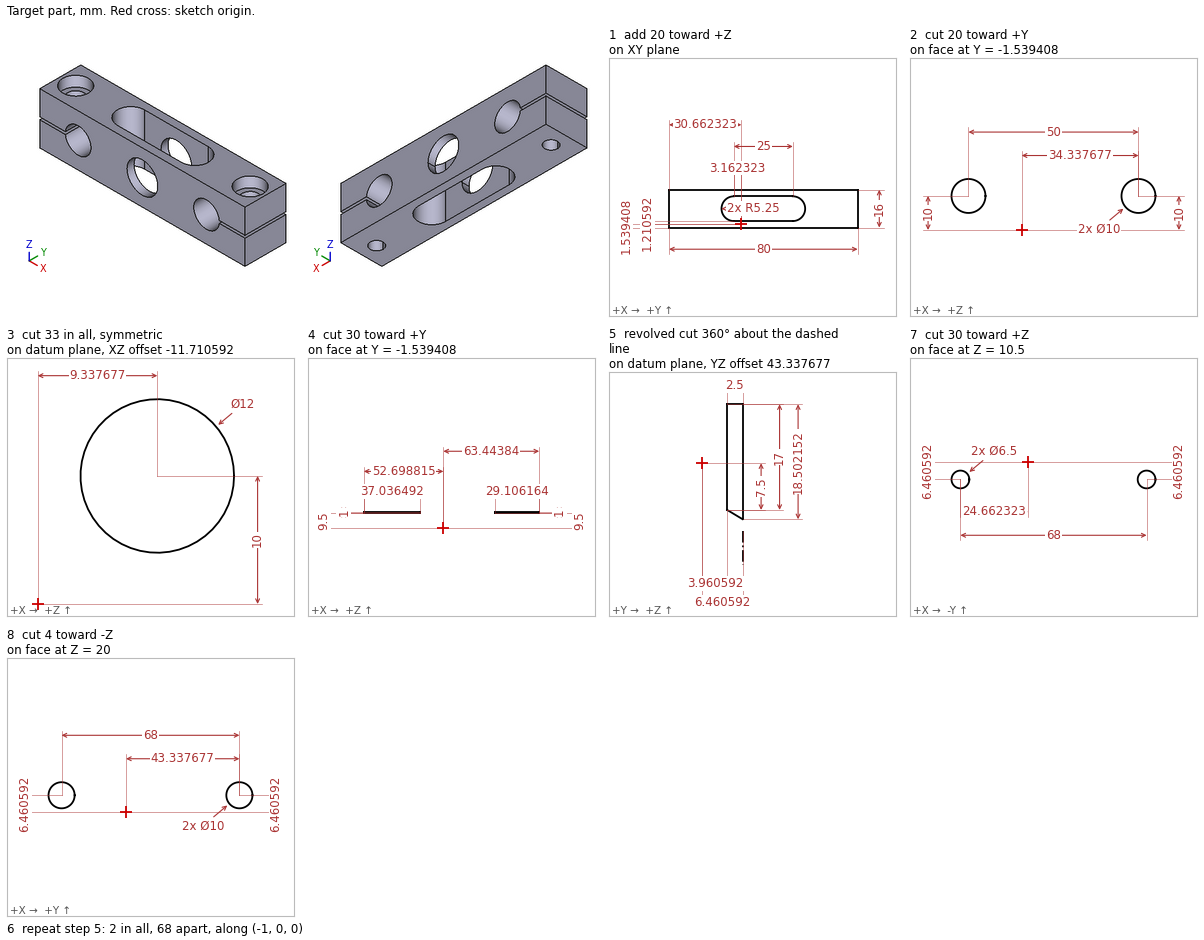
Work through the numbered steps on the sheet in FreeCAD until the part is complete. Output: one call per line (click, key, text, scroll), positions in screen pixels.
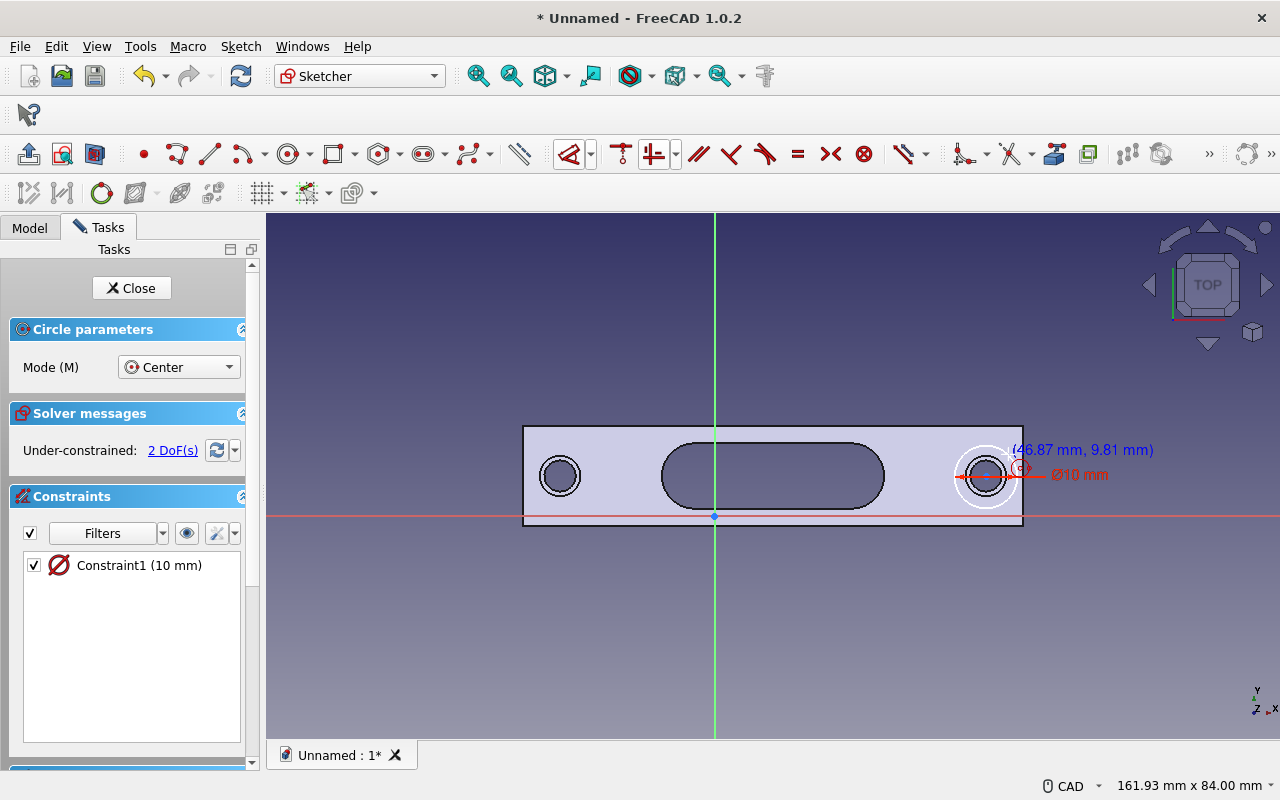
click(560, 476)
move(582, 454)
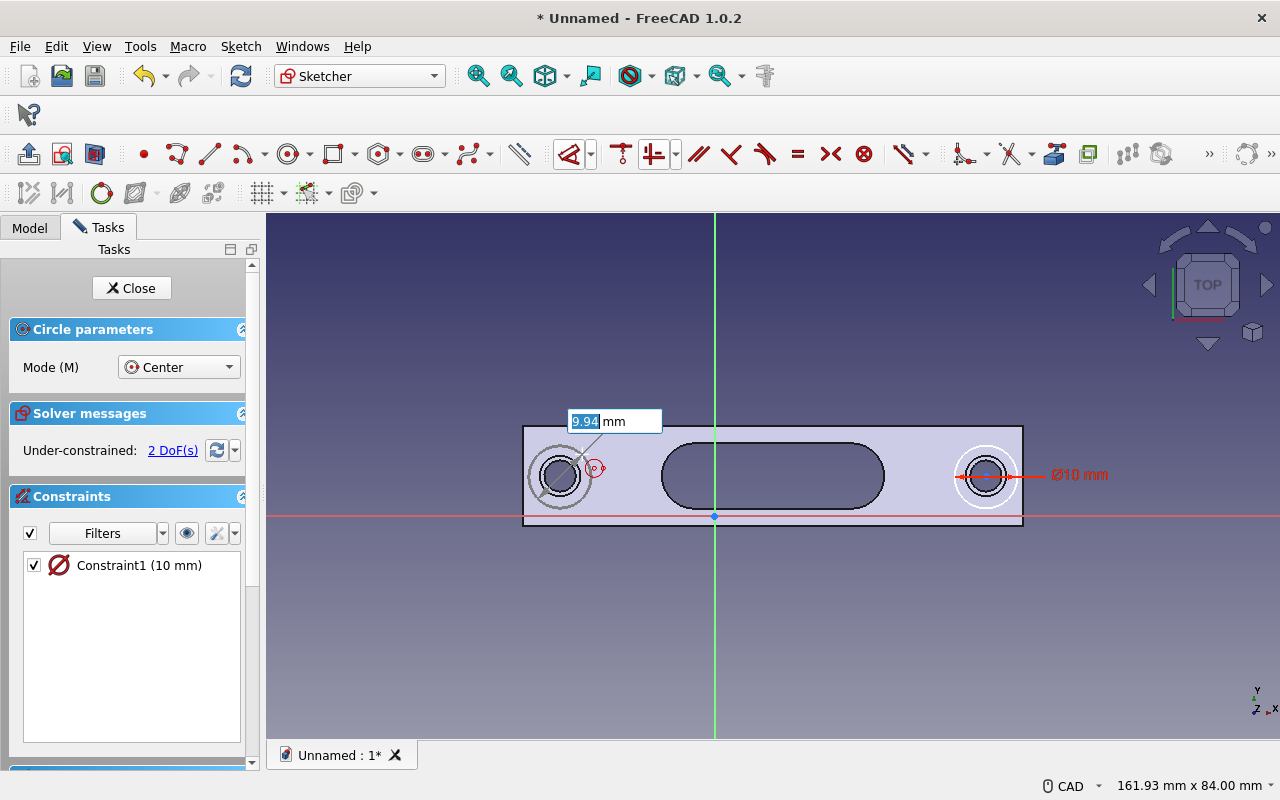
text(10)
key(Return)
key(Escape)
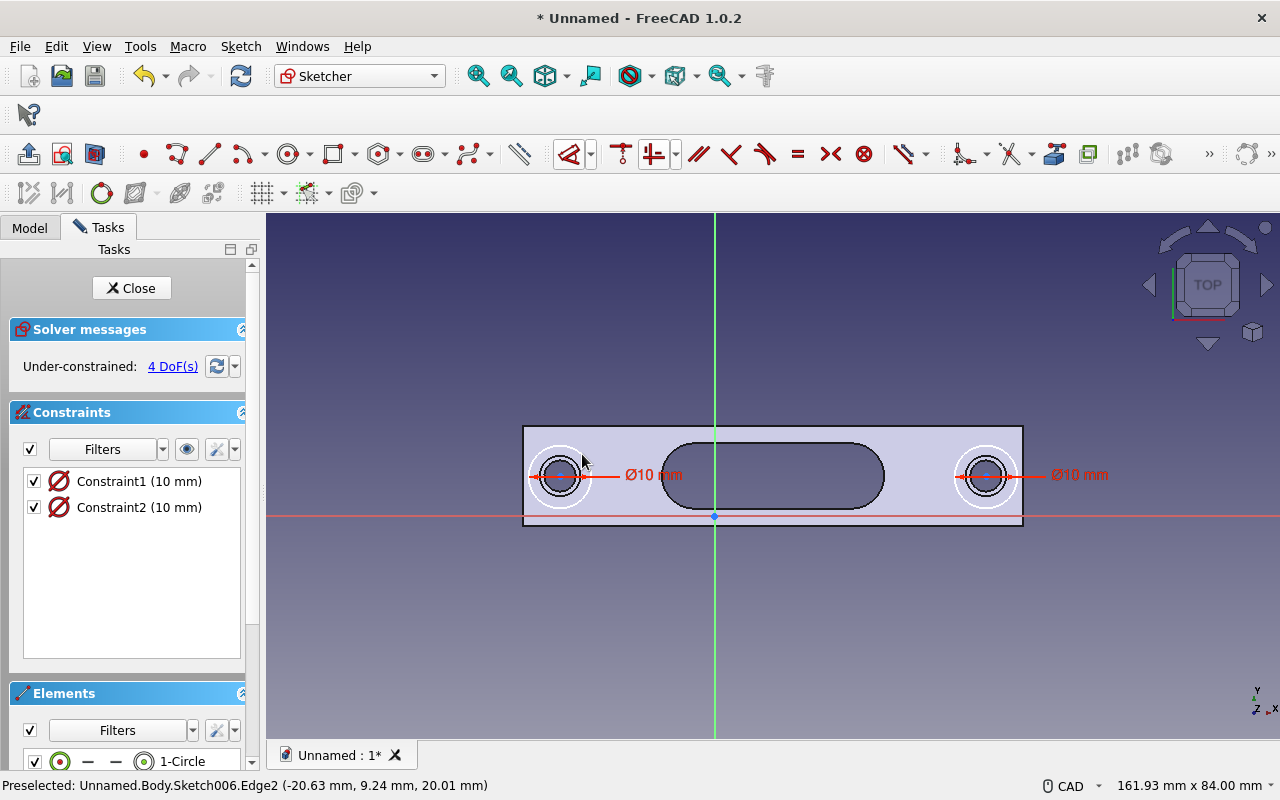
click(986, 477)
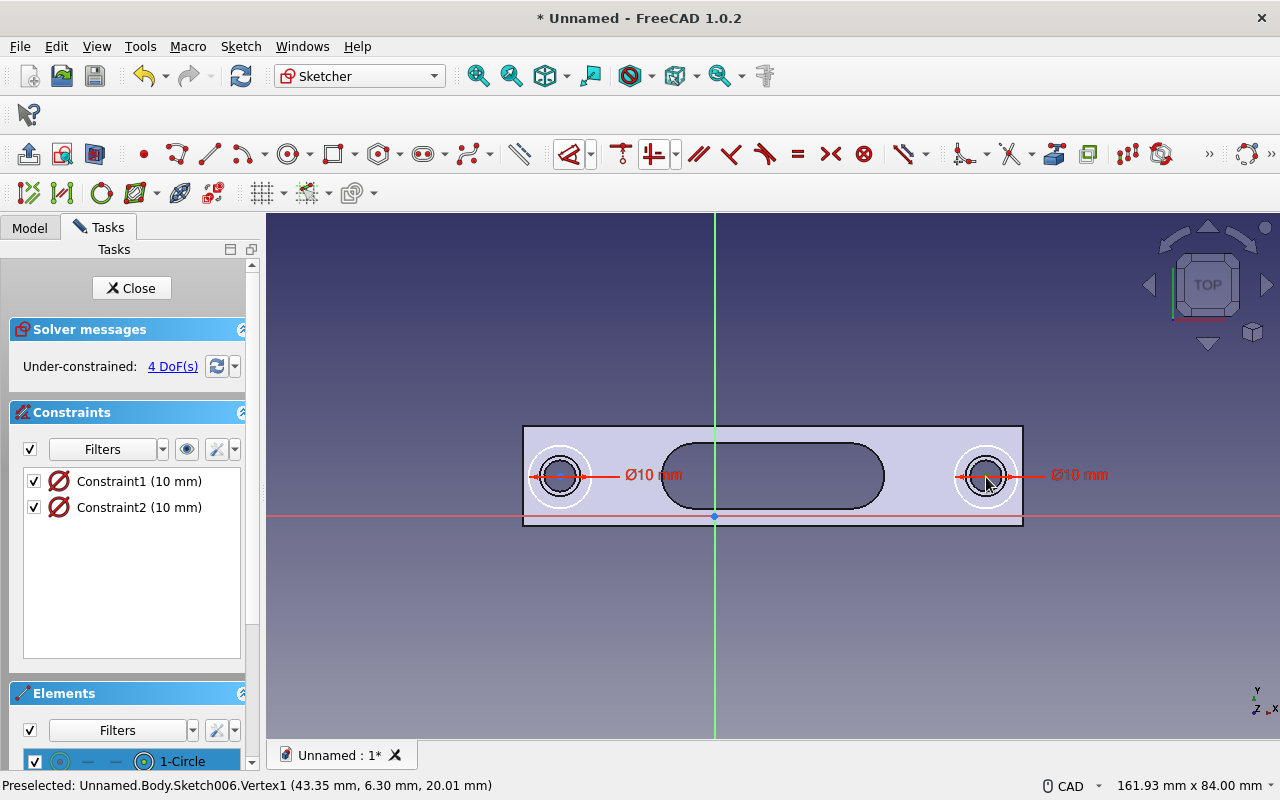
click(560, 477)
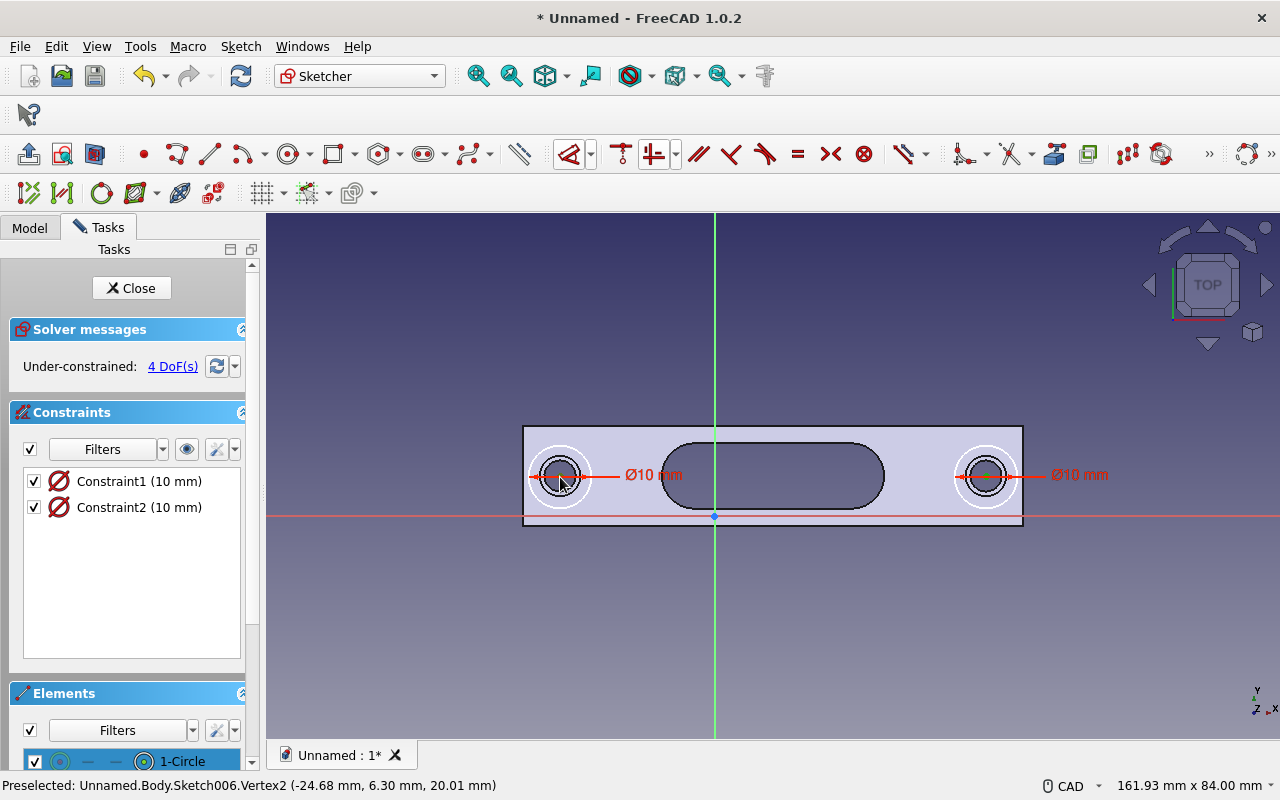
key(l)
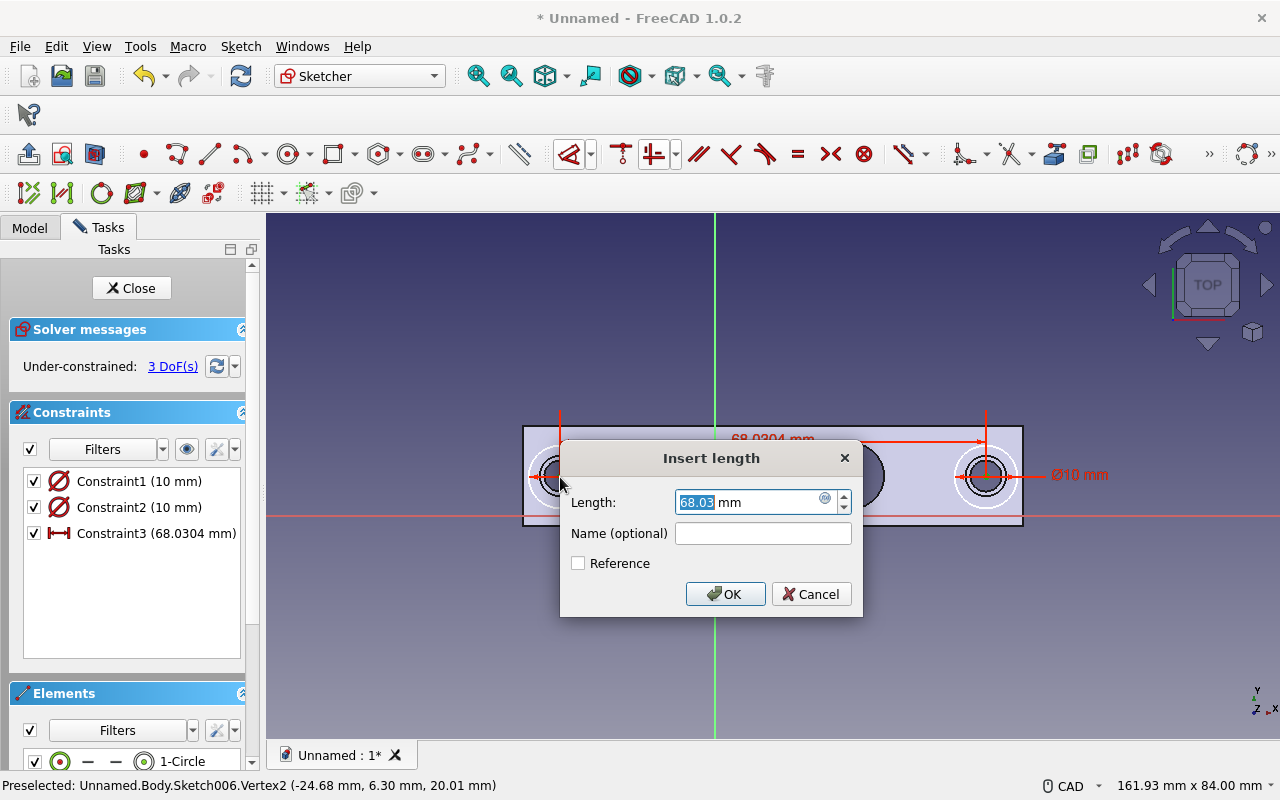
text(68)
key(Return)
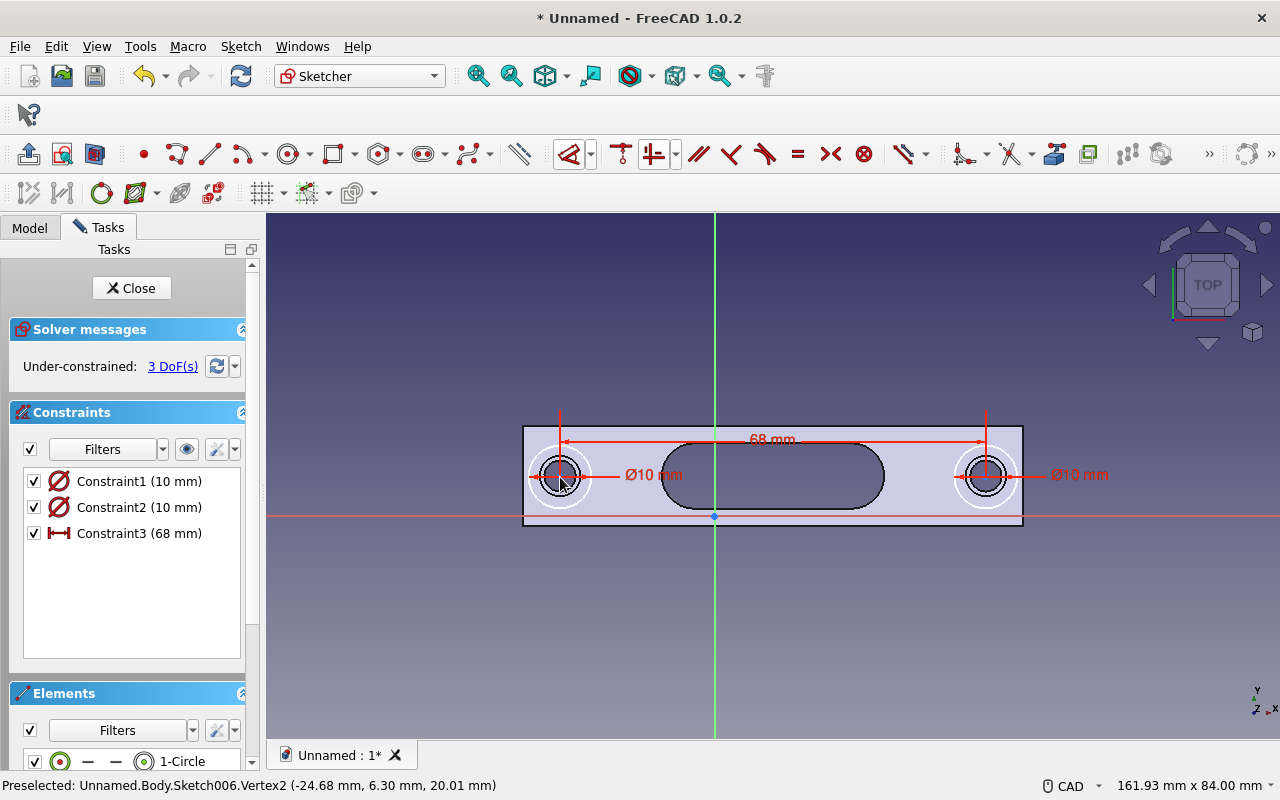
click(986, 477)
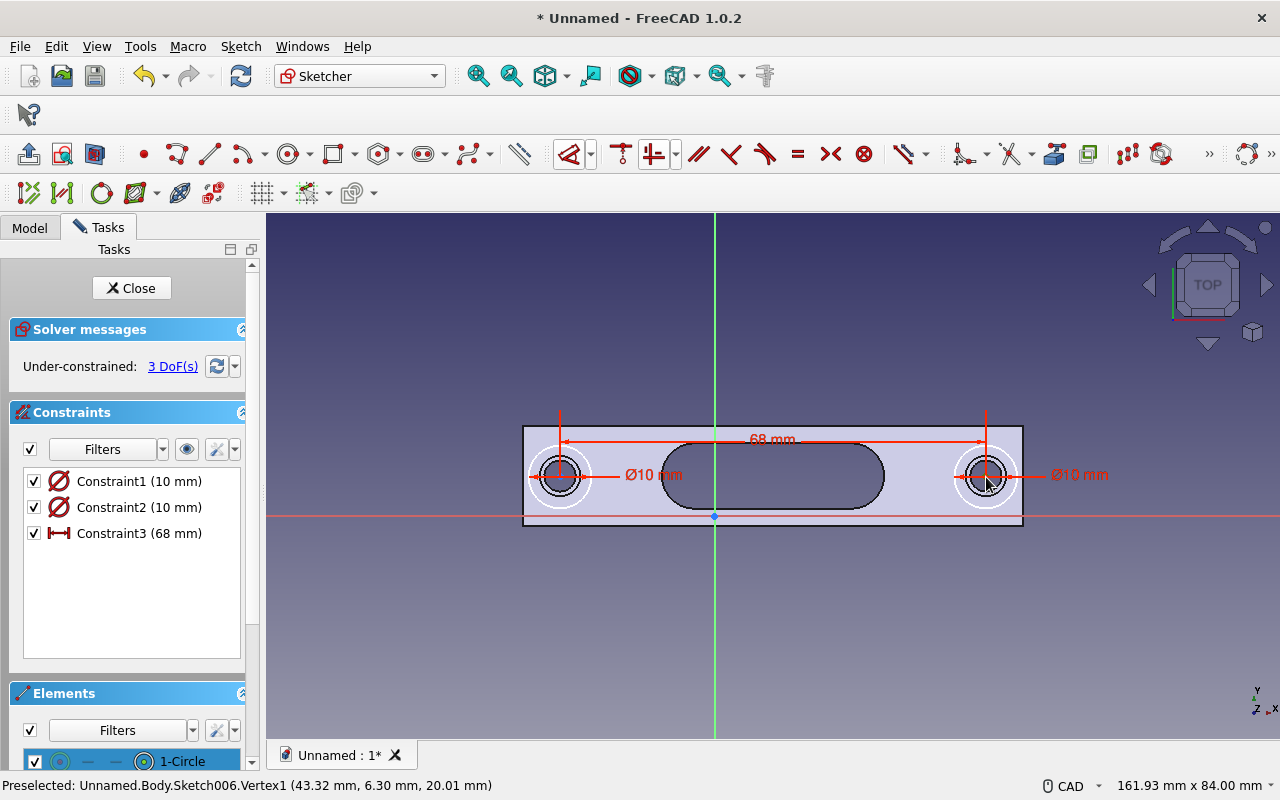
key(i)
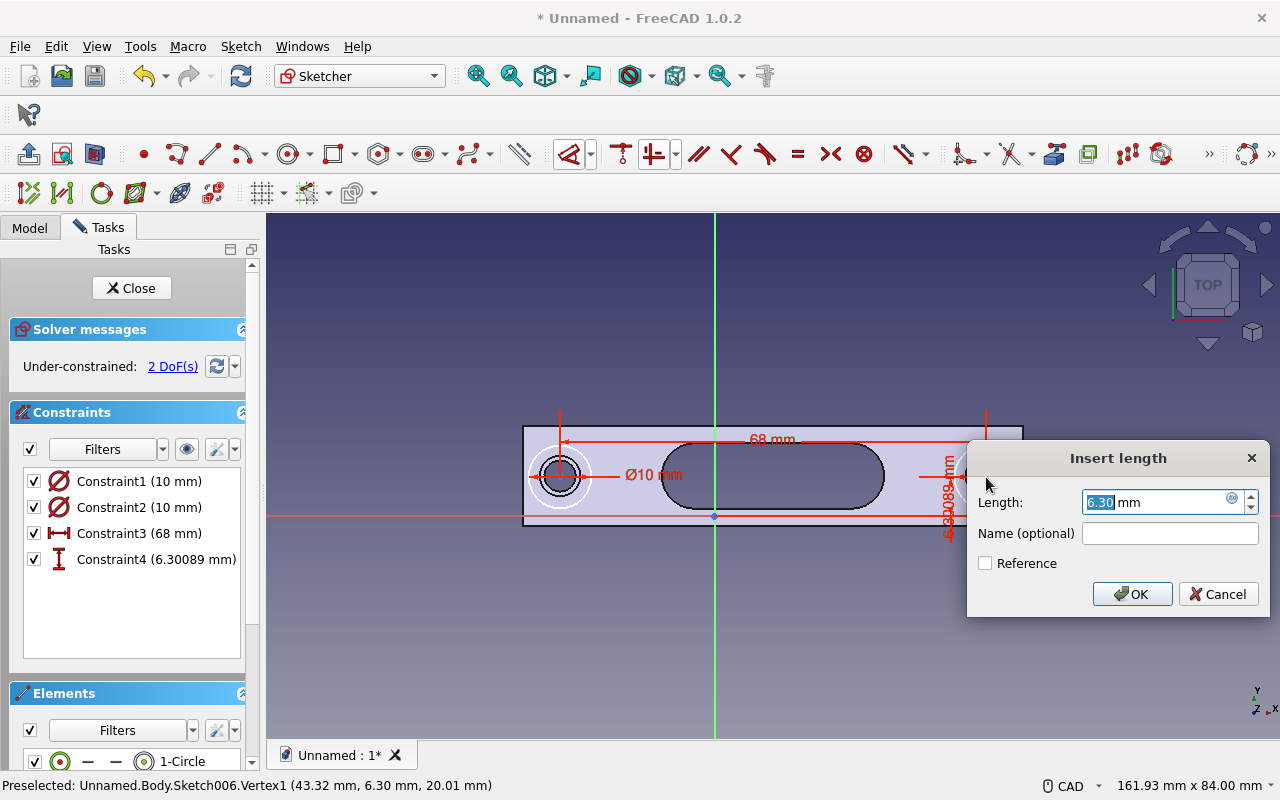
text(6.460592)
key(Return)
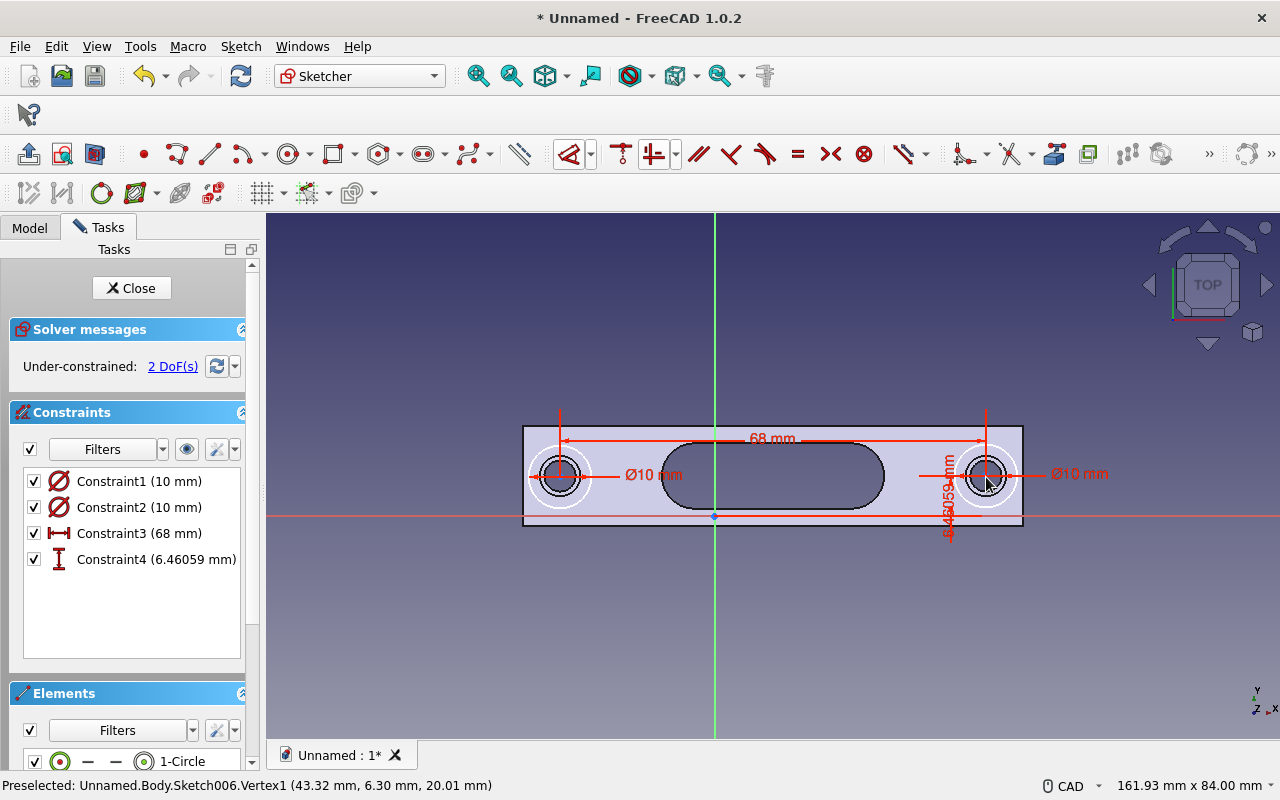
click(560, 477)